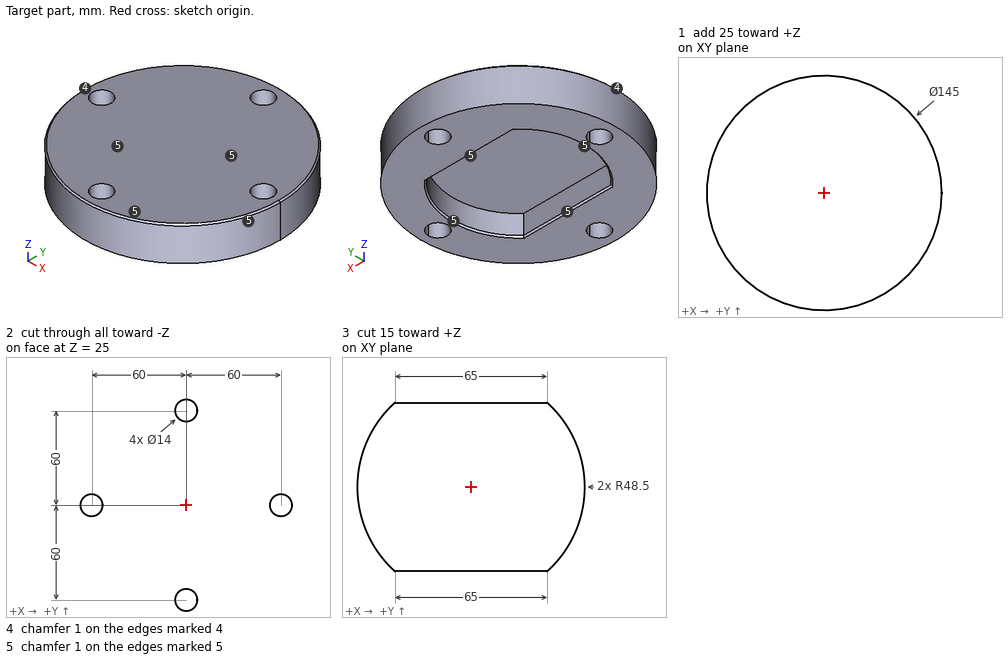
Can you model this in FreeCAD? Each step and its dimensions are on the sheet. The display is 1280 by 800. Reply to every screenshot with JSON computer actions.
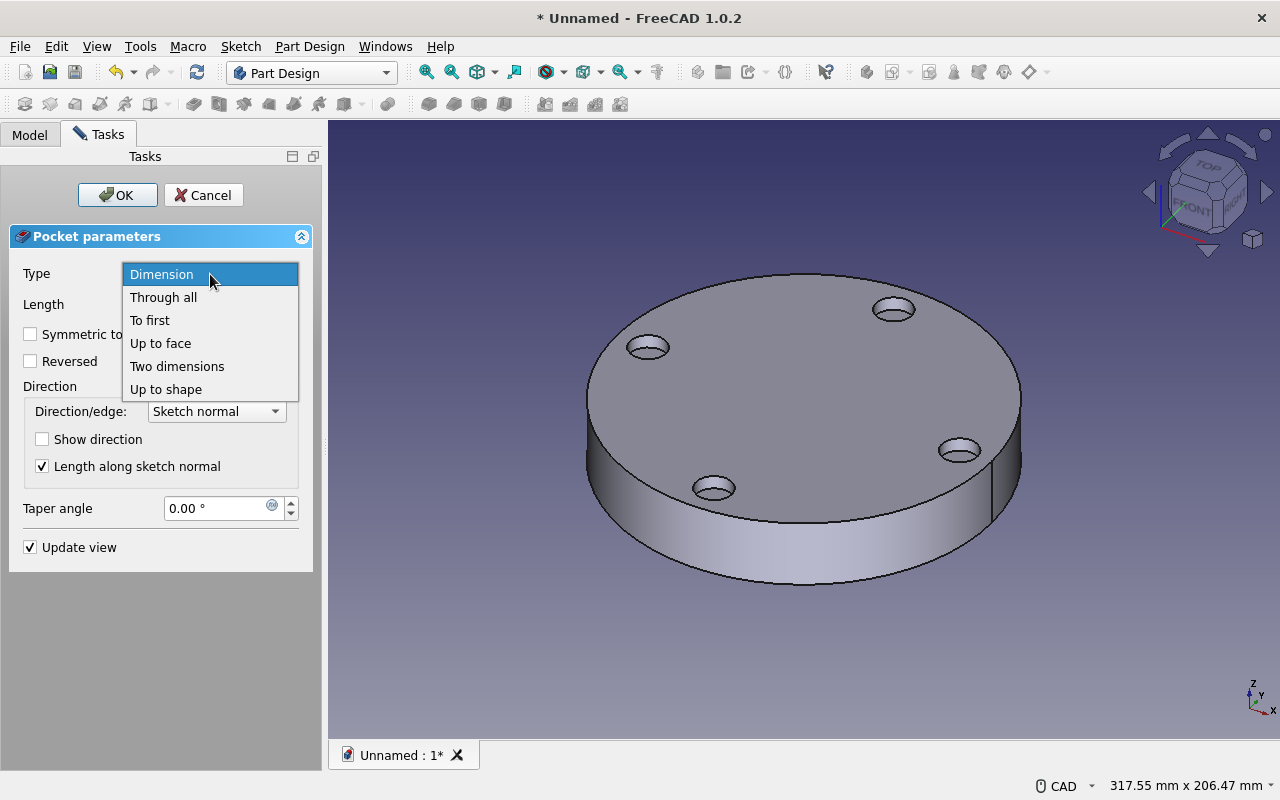
{"action": "left_click", "coordinate": [208, 298]}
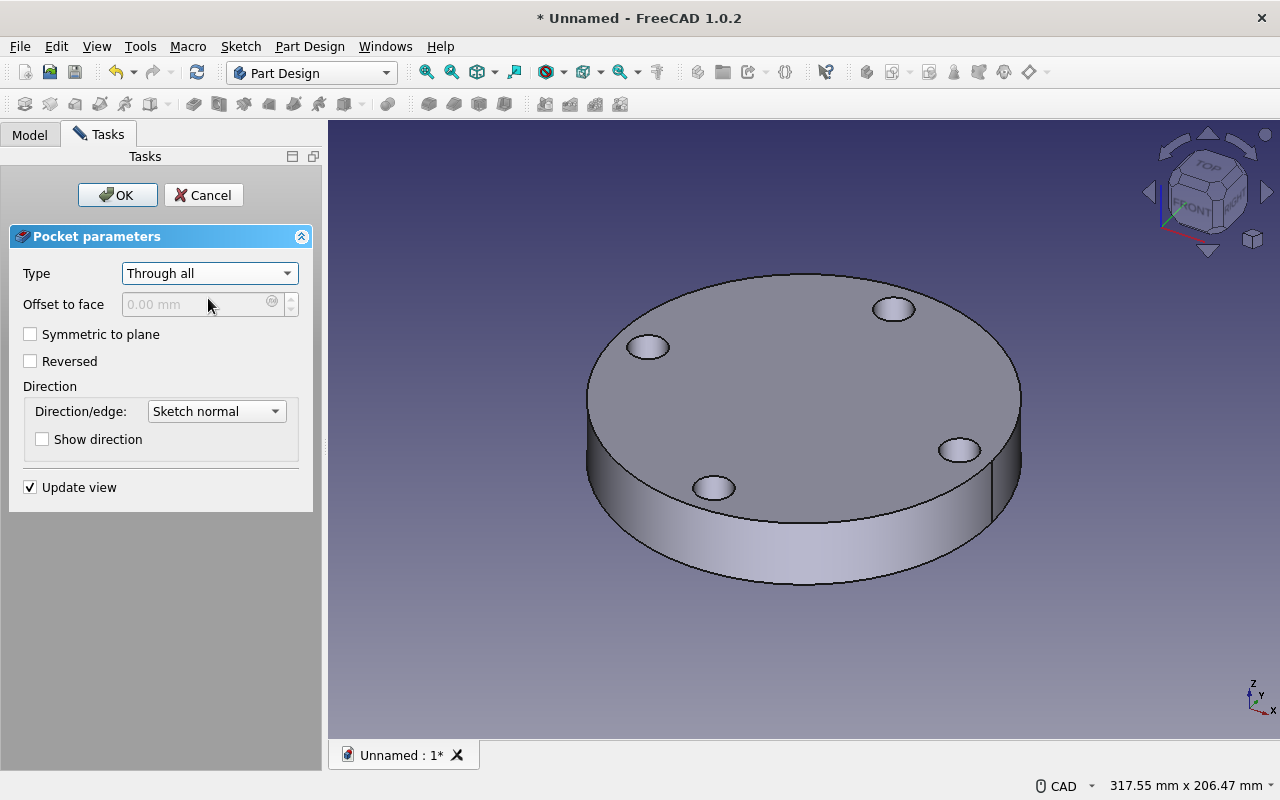
{"action": "left_click", "coordinate": [118, 195]}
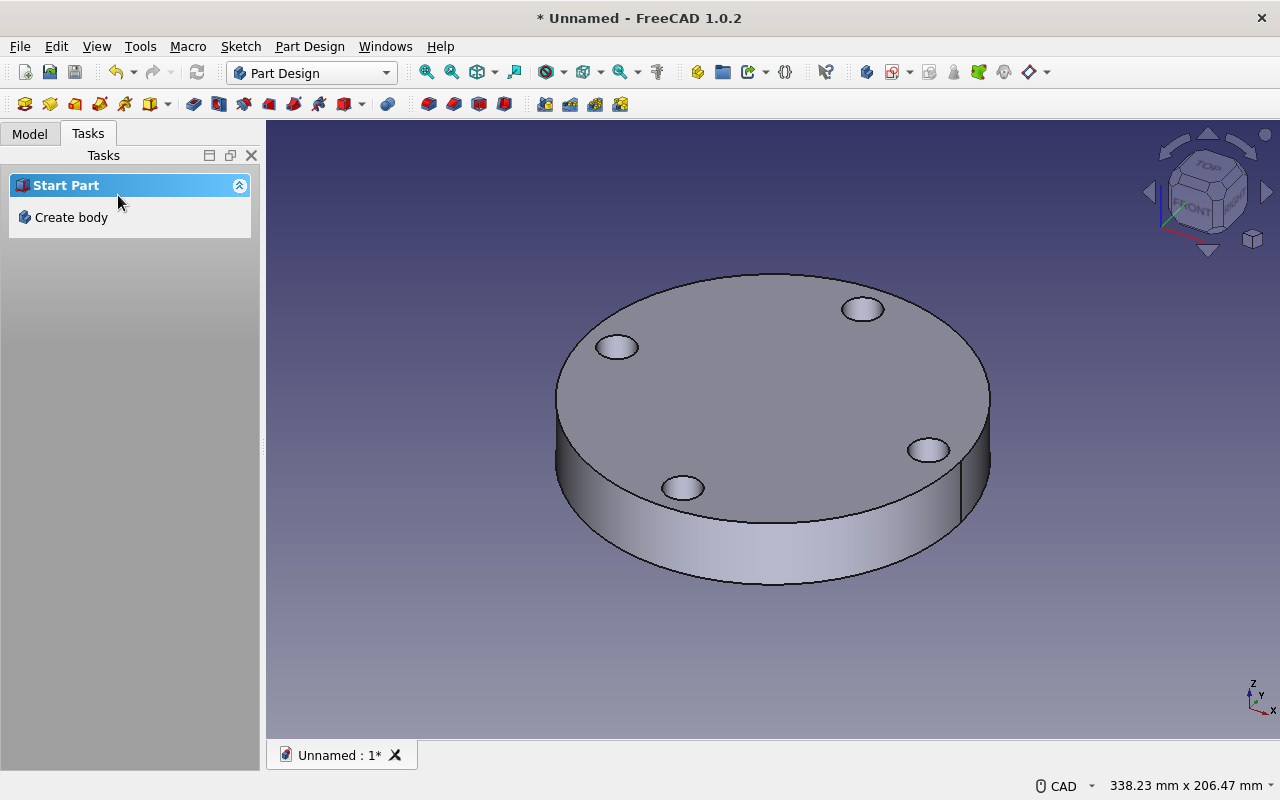
{"action": "left_click", "coordinate": [892, 72]}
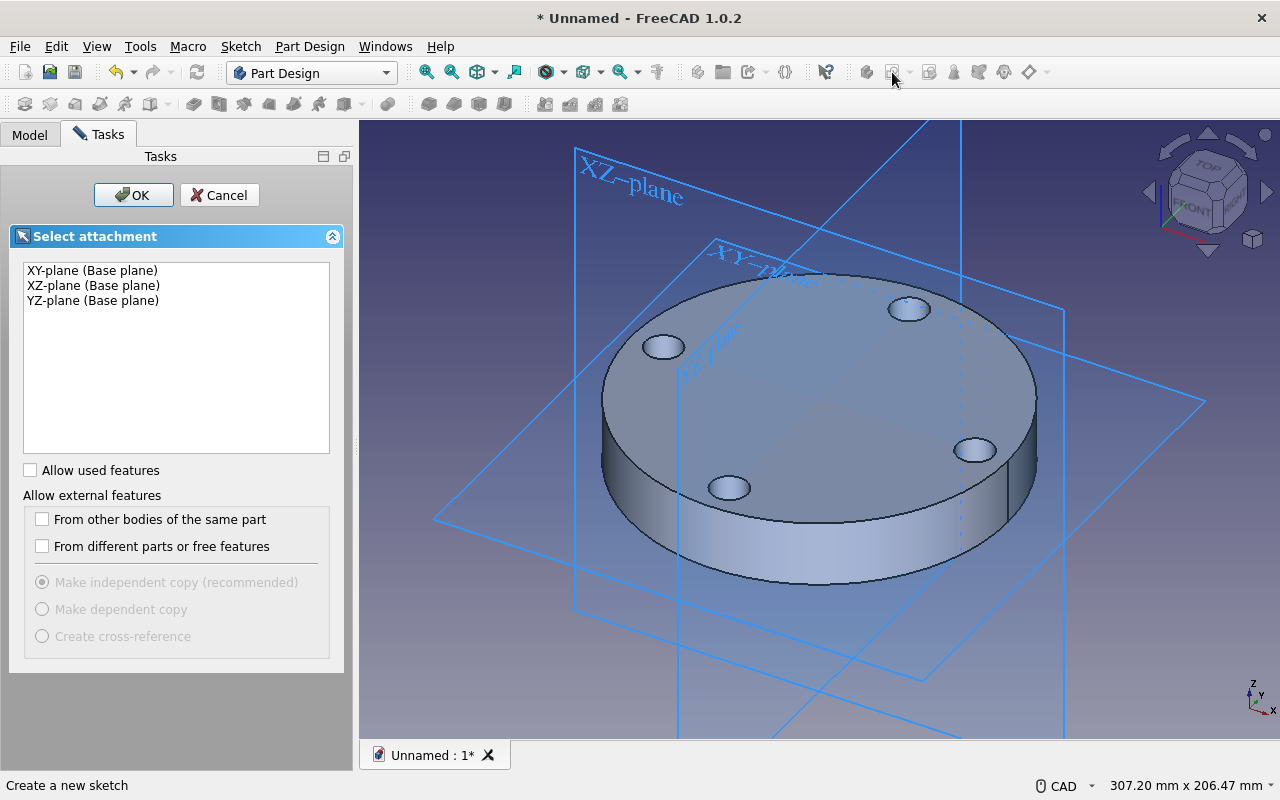
{"action": "left_click", "coordinate": [84, 270]}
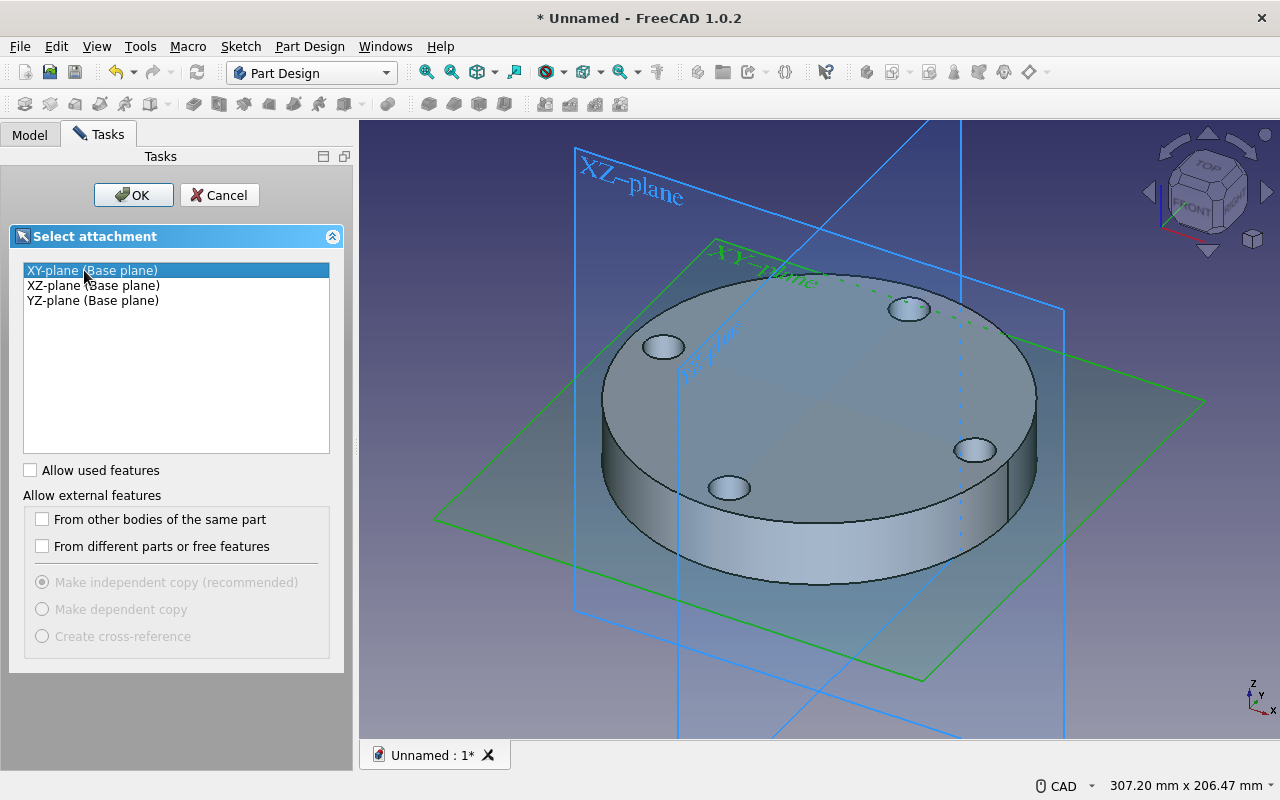
{"action": "left_click", "coordinate": [134, 195]}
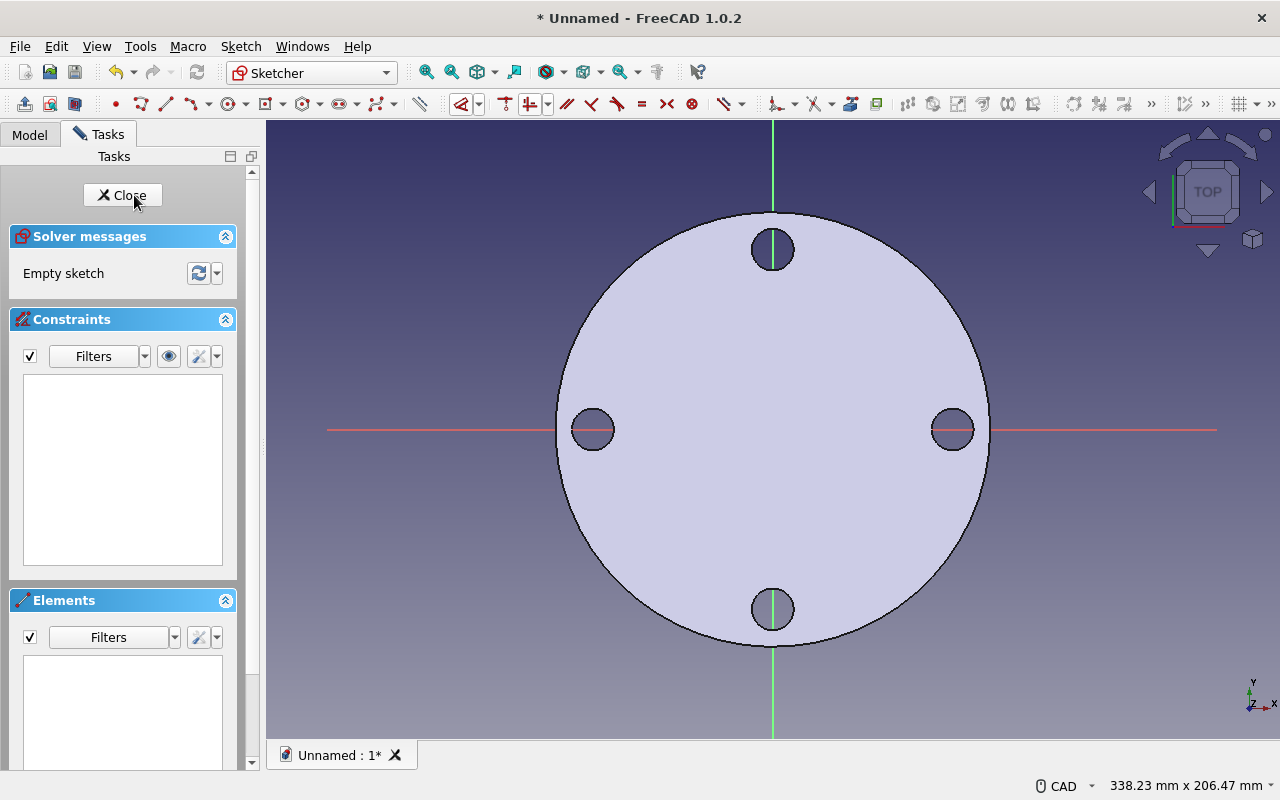
{"action": "left_click", "coordinate": [75, 104]}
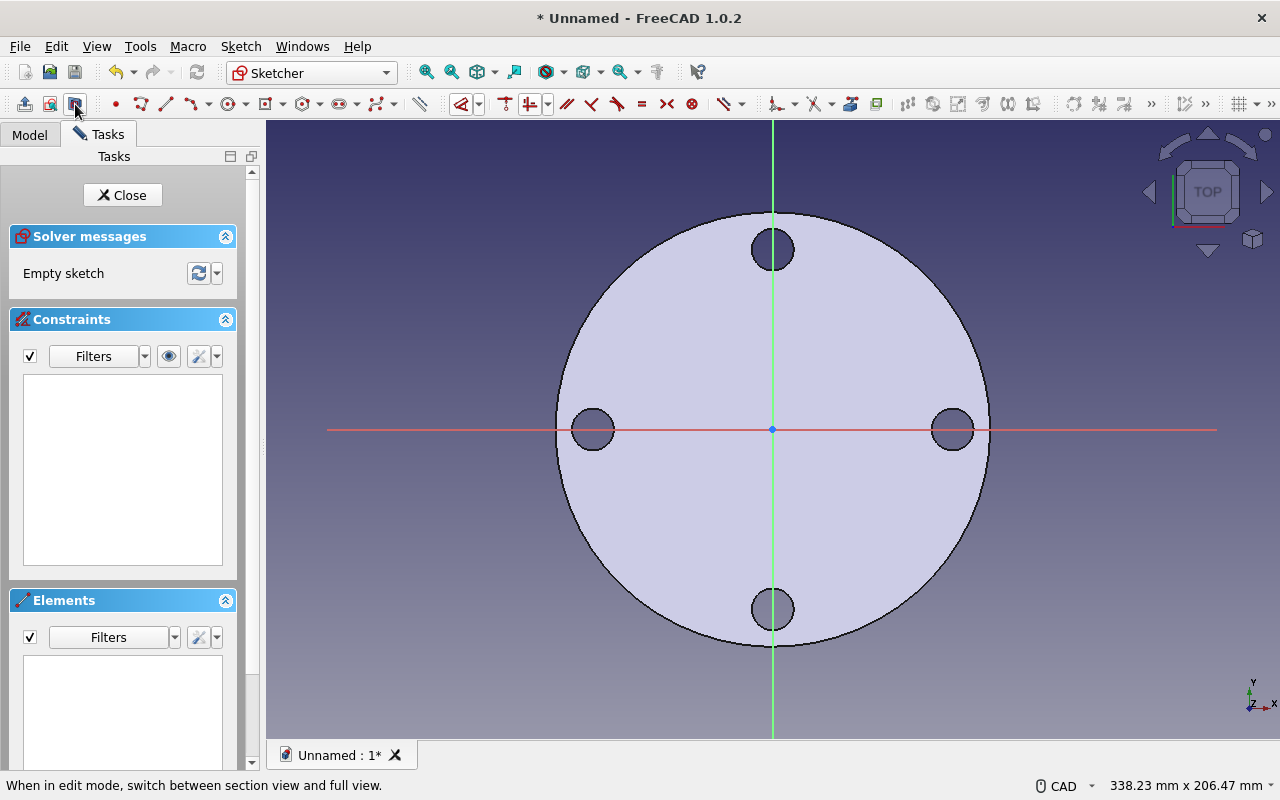
{"action": "scroll", "coordinate": [856, 430], "scroll_direction": "up", "scroll_amount": 3}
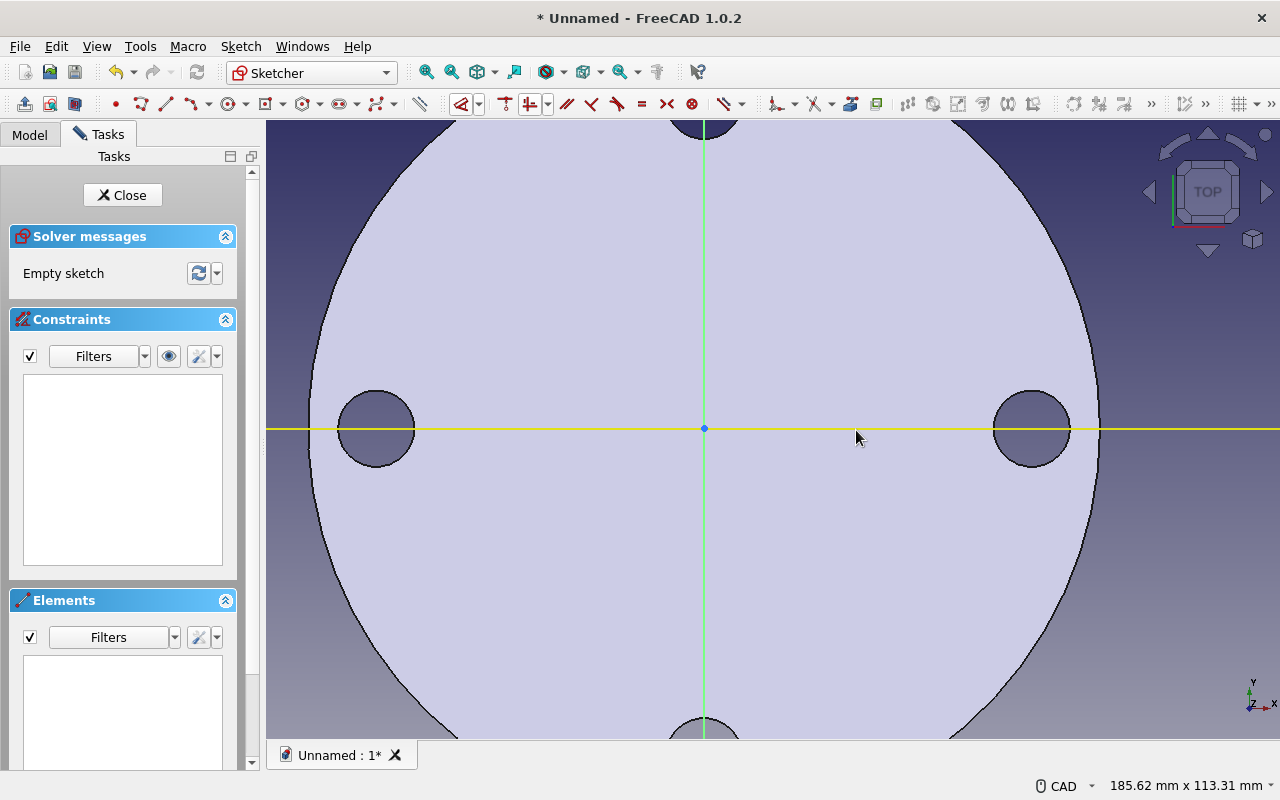
{"action": "left_click", "coordinate": [166, 104]}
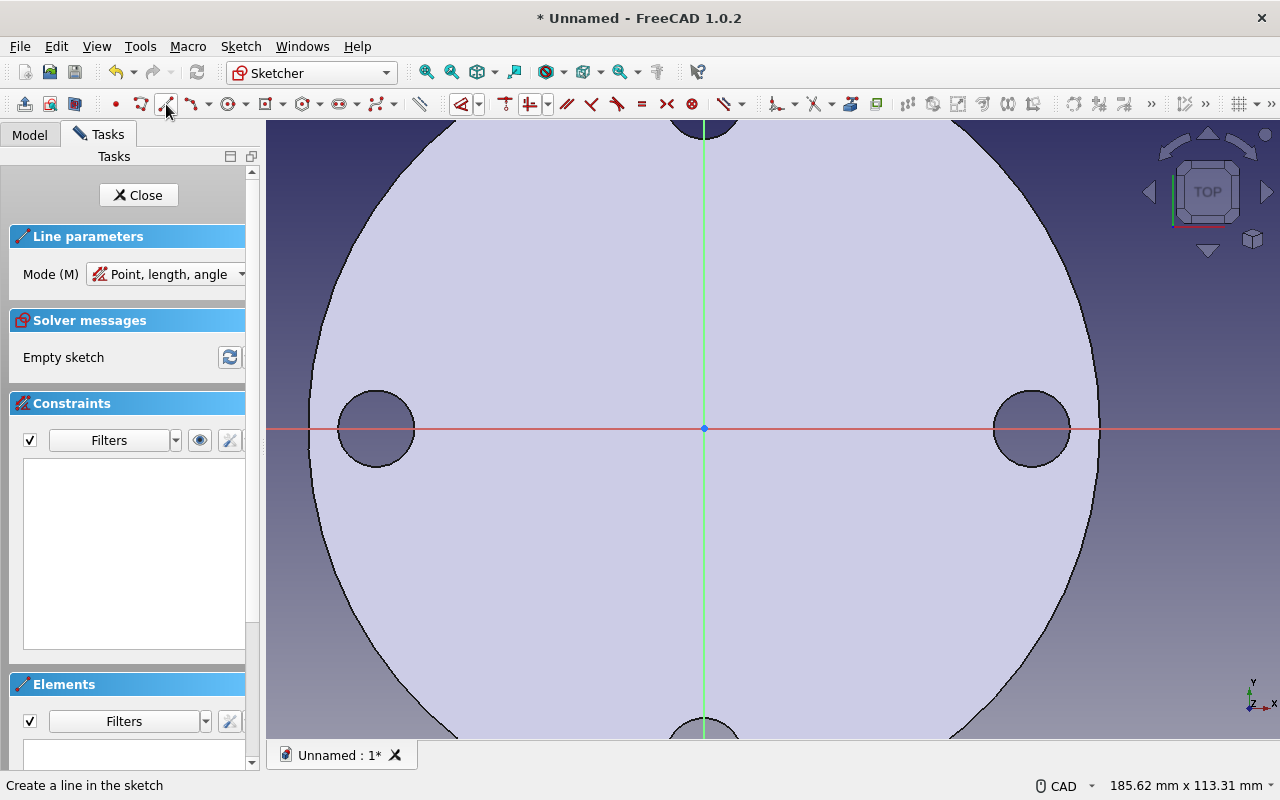
{"action": "left_click", "coordinate": [526, 232]}
{"action": "left_click", "coordinate": [882, 232]}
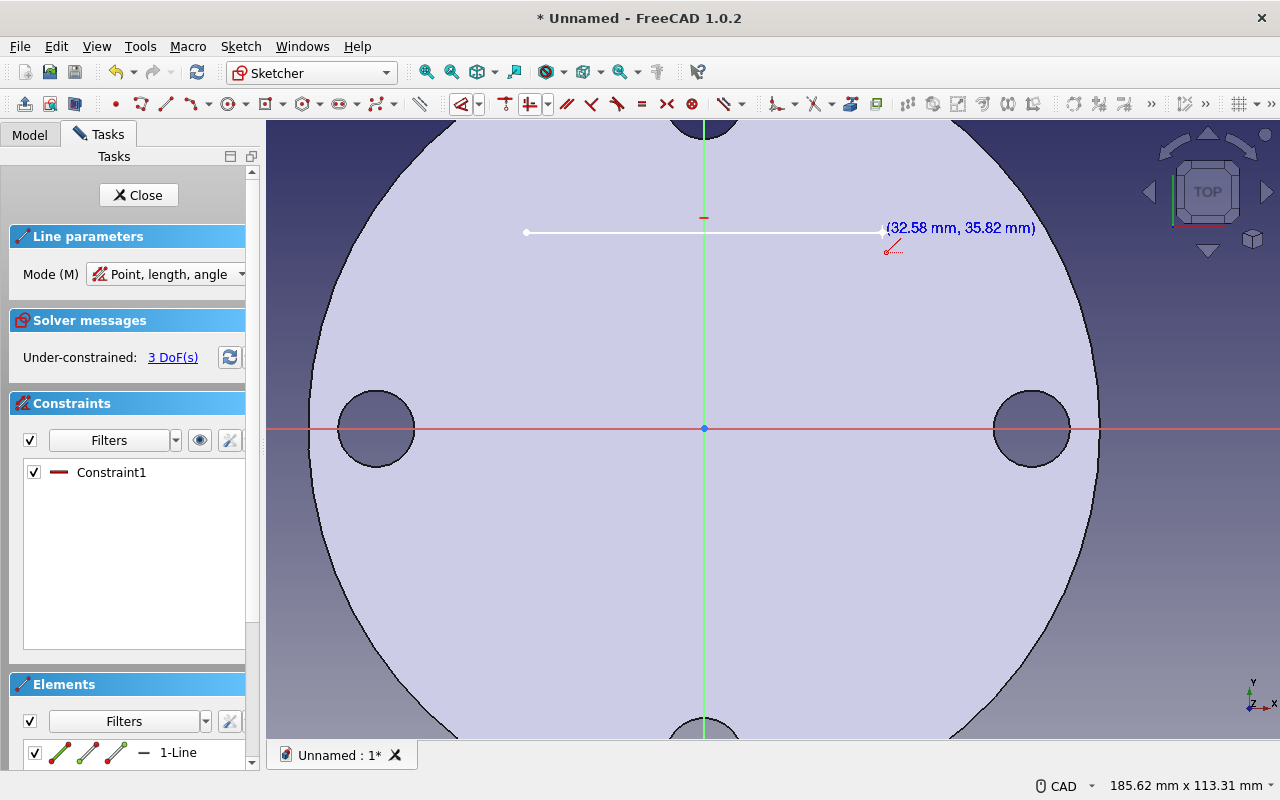
{"action": "left_click", "coordinate": [882, 625]}
{"action": "left_click", "coordinate": [526, 625]}